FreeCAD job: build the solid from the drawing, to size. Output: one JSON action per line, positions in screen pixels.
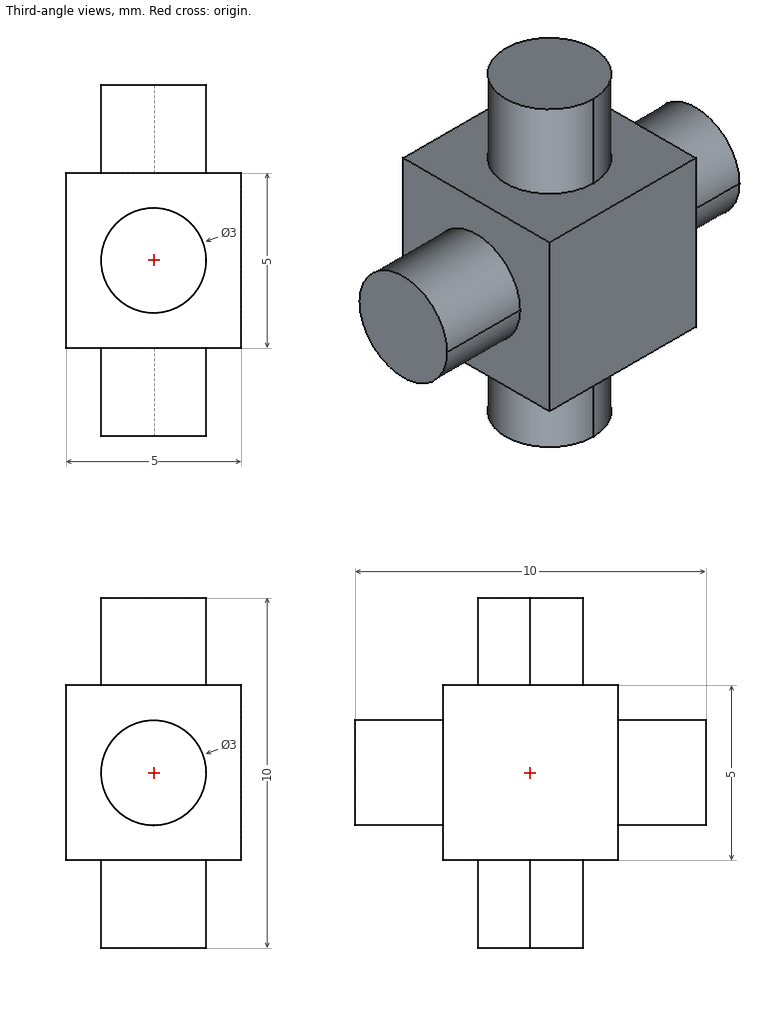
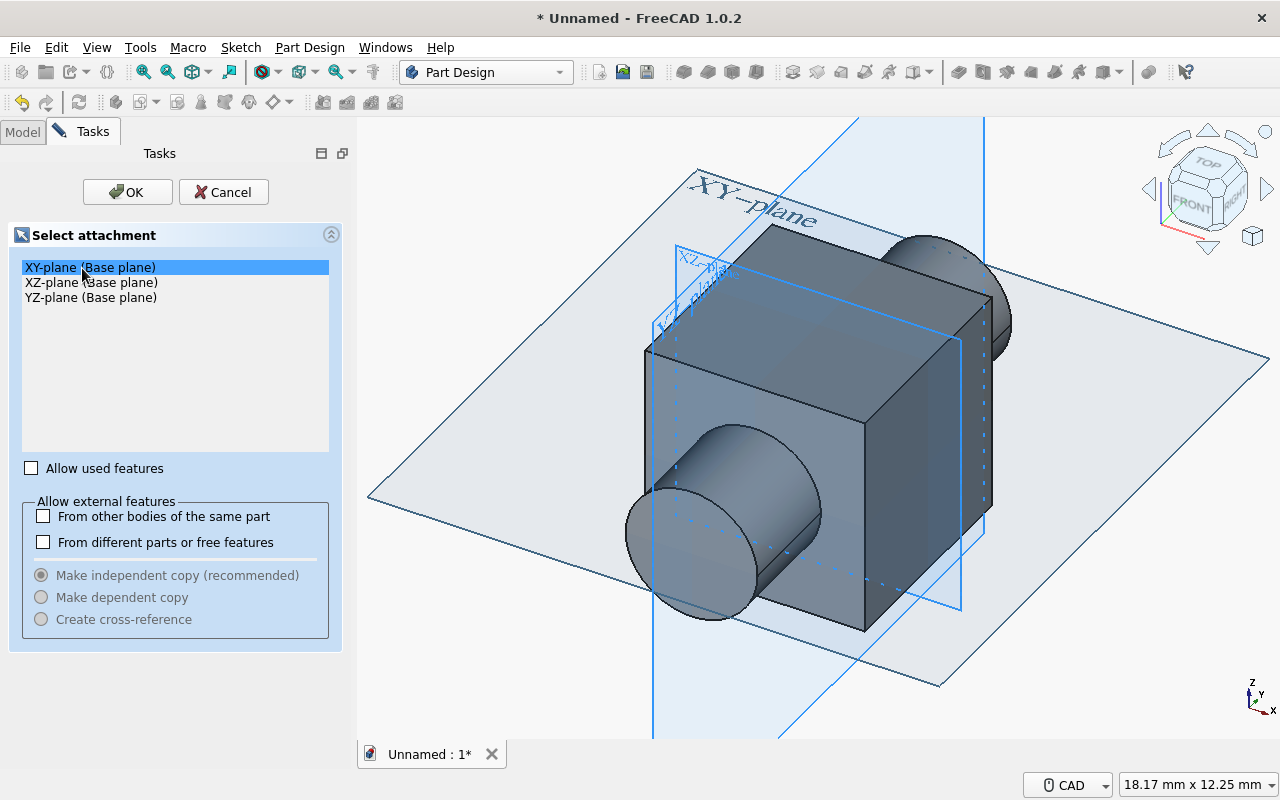
{"action": "left_click", "coordinate": [128, 192]}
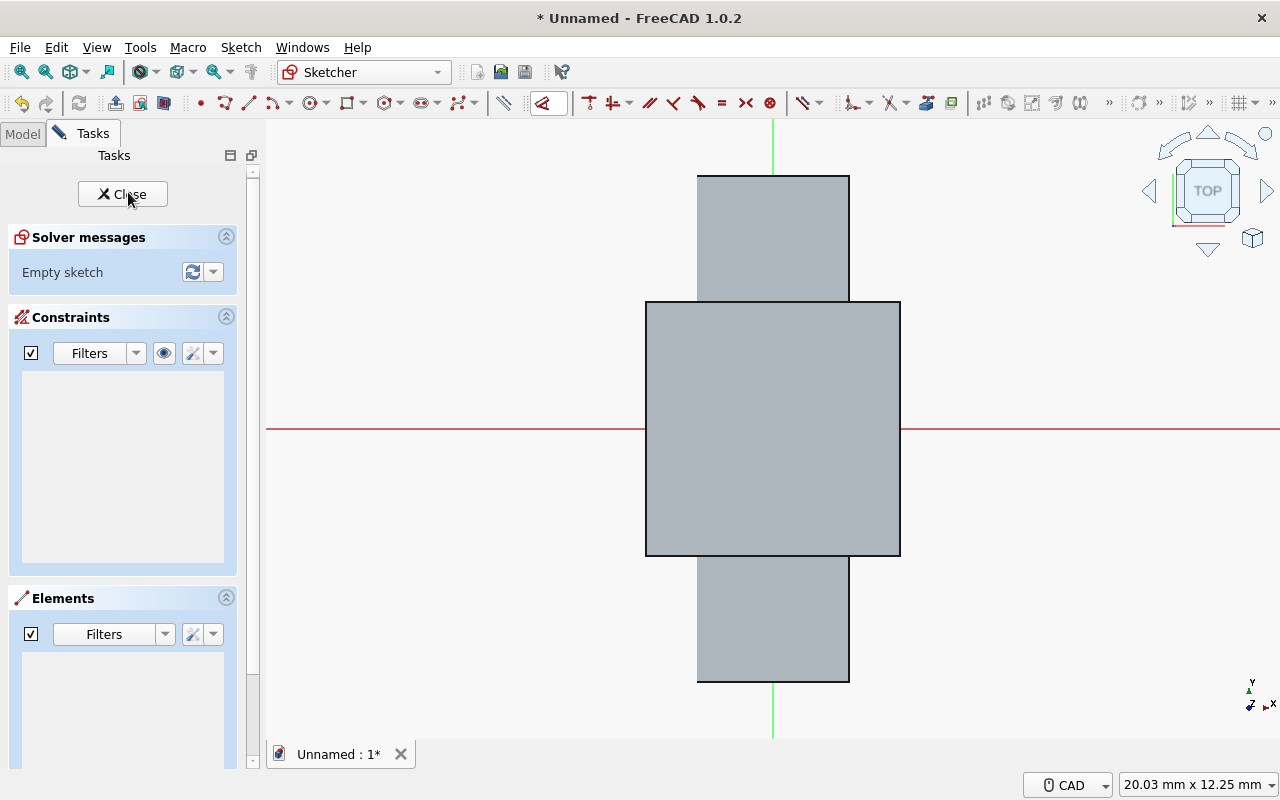
{"action": "left_click", "coordinate": [164, 104]}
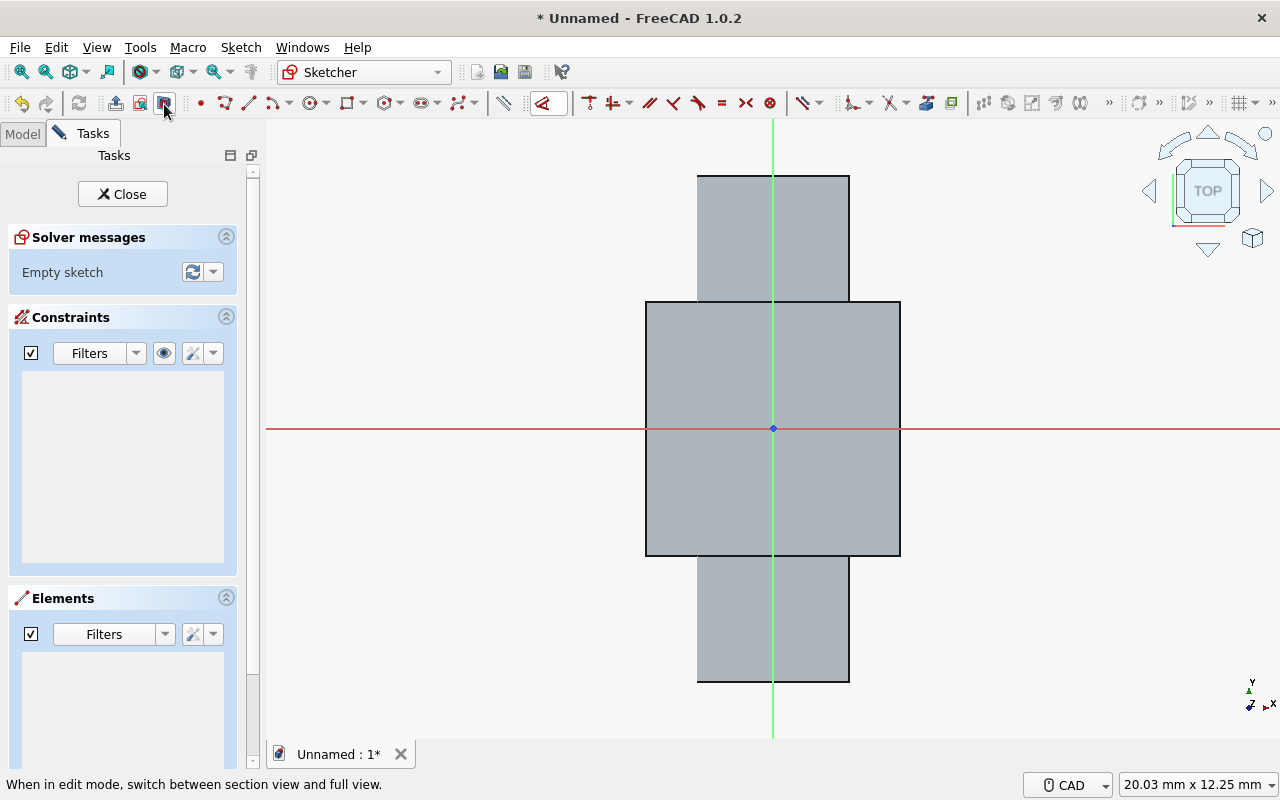
{"action": "scroll", "coordinate": [813, 429], "scroll_direction": "up", "scroll_amount": 5}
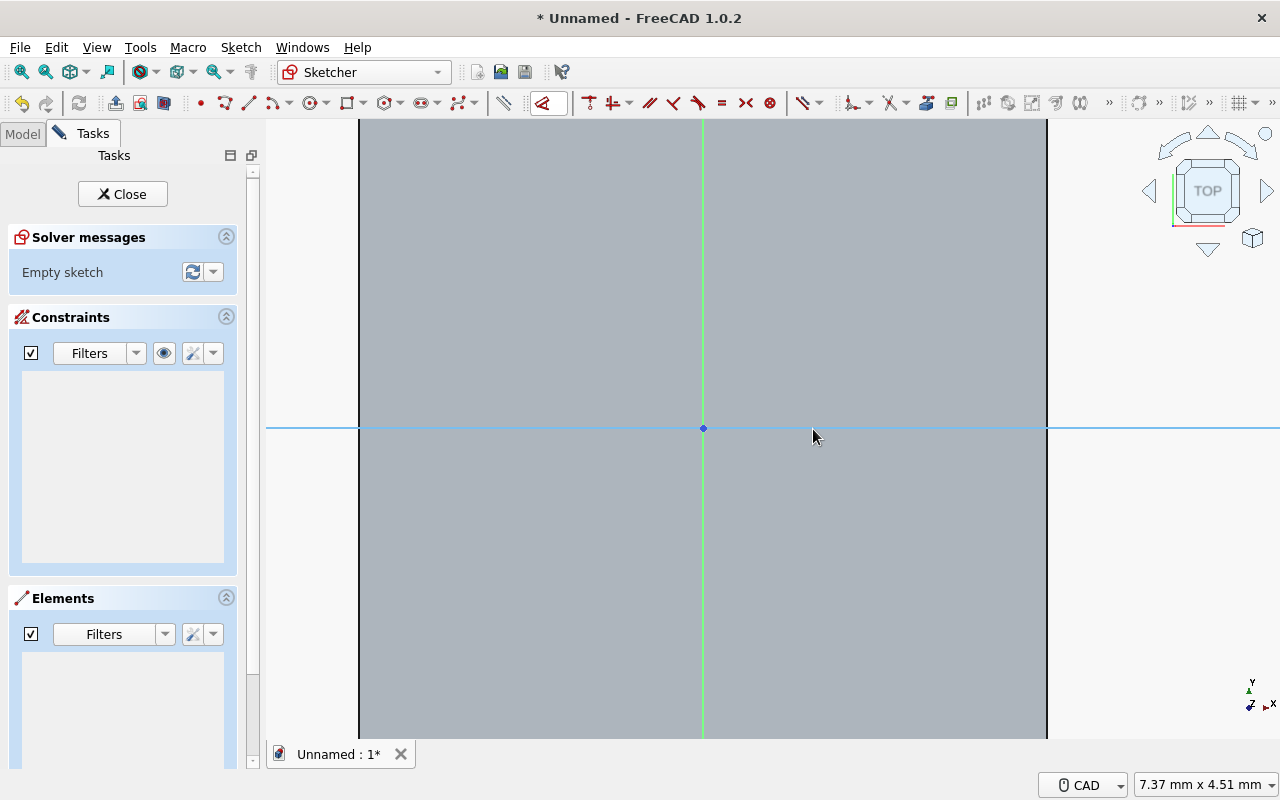
{"action": "left_click", "coordinate": [310, 104]}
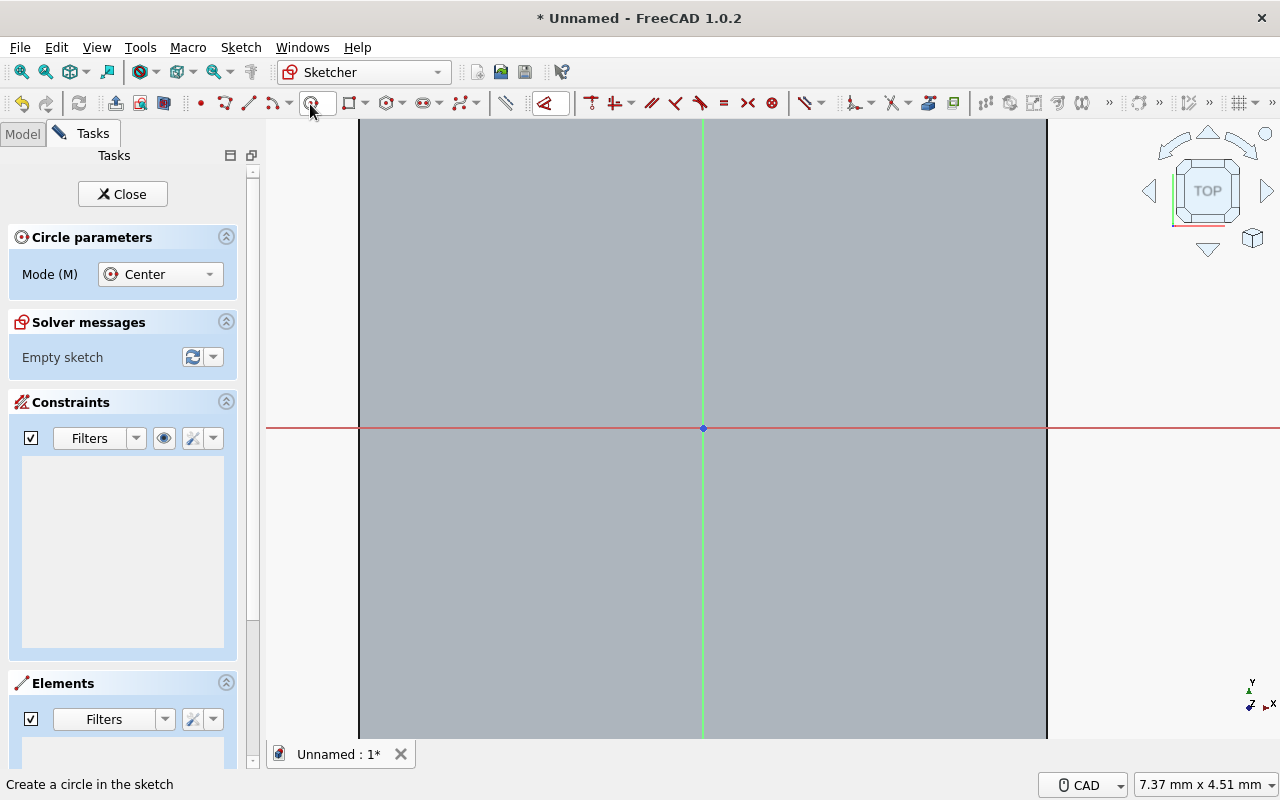
{"action": "left_click", "coordinate": [703, 428]}
{"action": "mouse_move", "coordinate": [849, 282]}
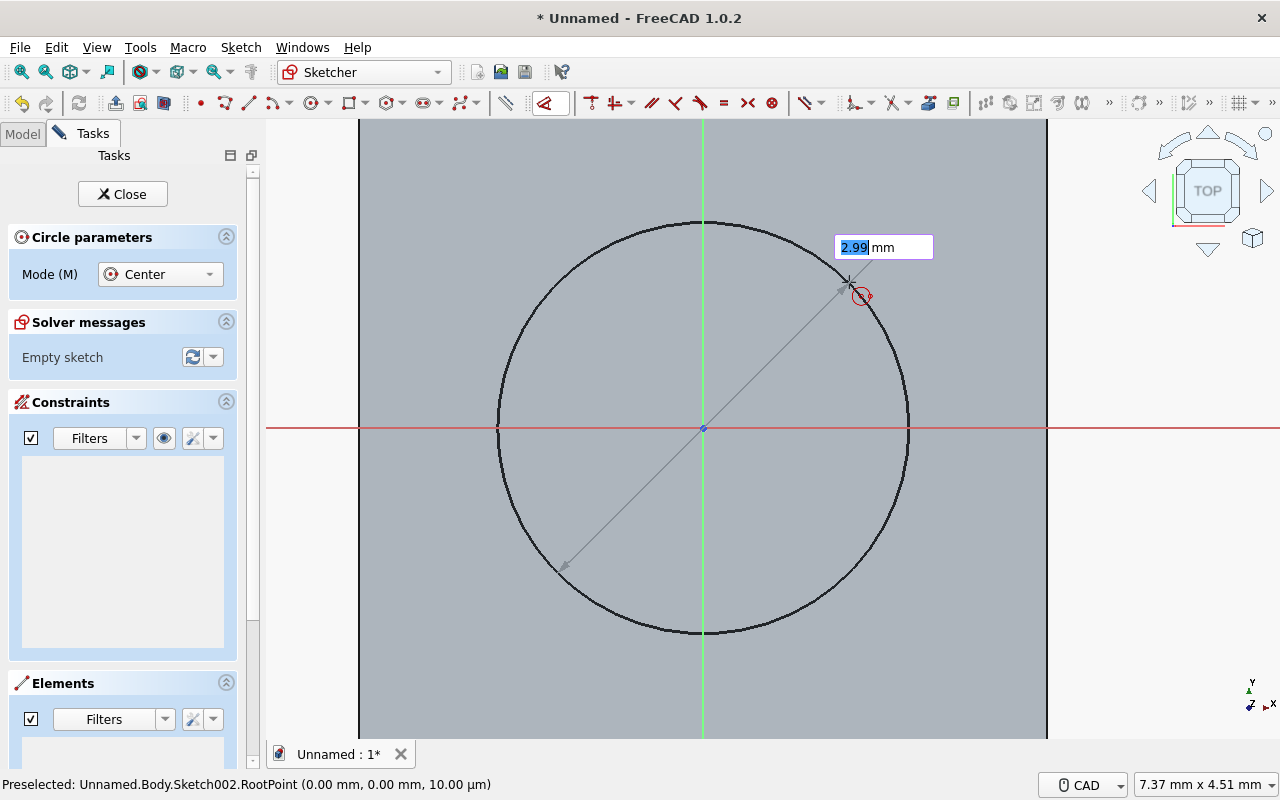
{"action": "type", "text": "3"}
{"action": "key", "text": "Return"}
{"action": "key", "text": "Escape"}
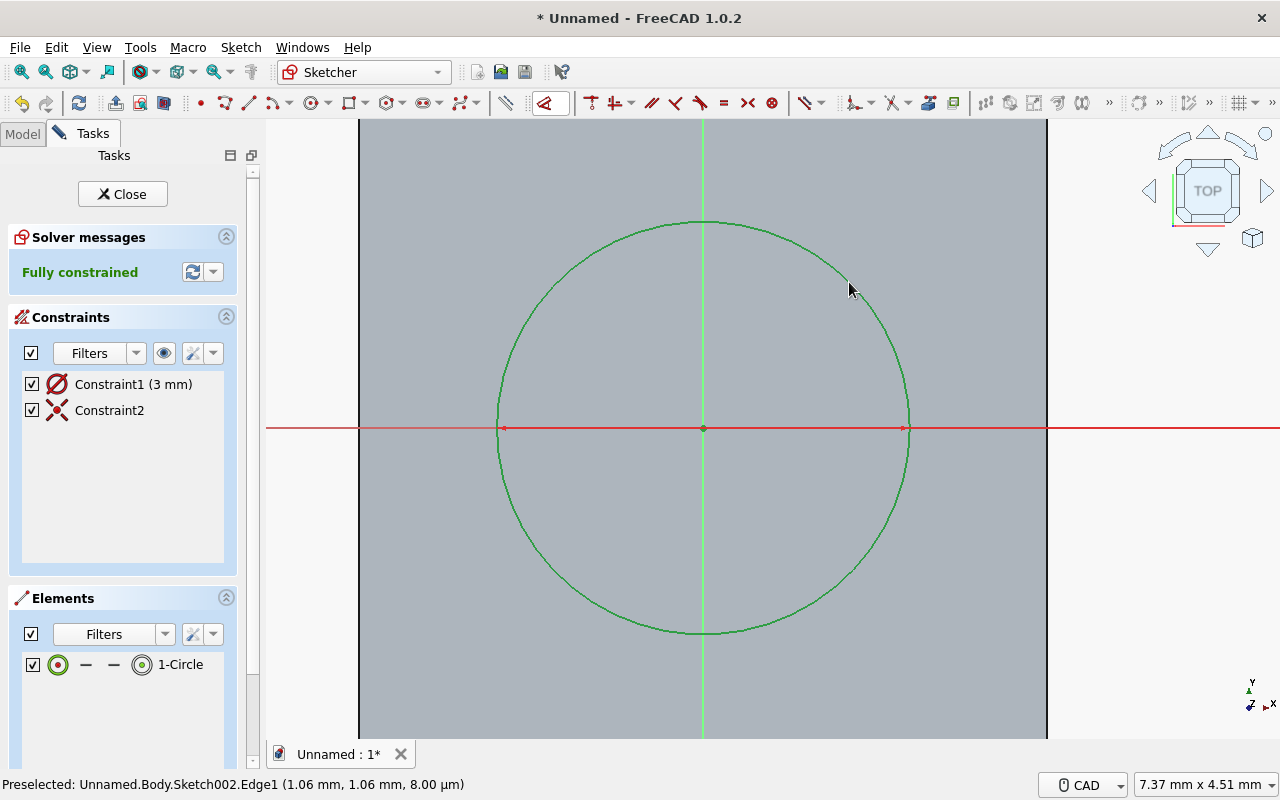
{"action": "left_click", "coordinate": [123, 194]}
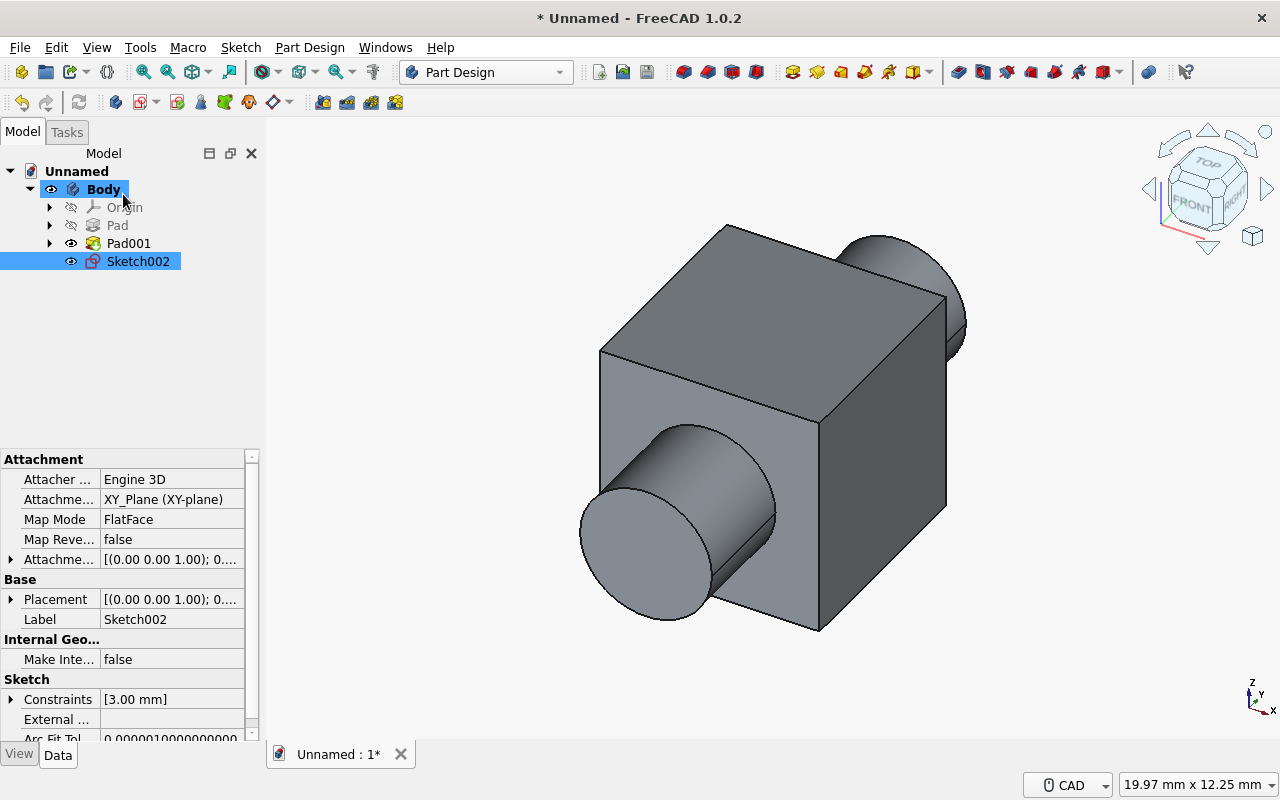
{"action": "left_click", "coordinate": [794, 72]}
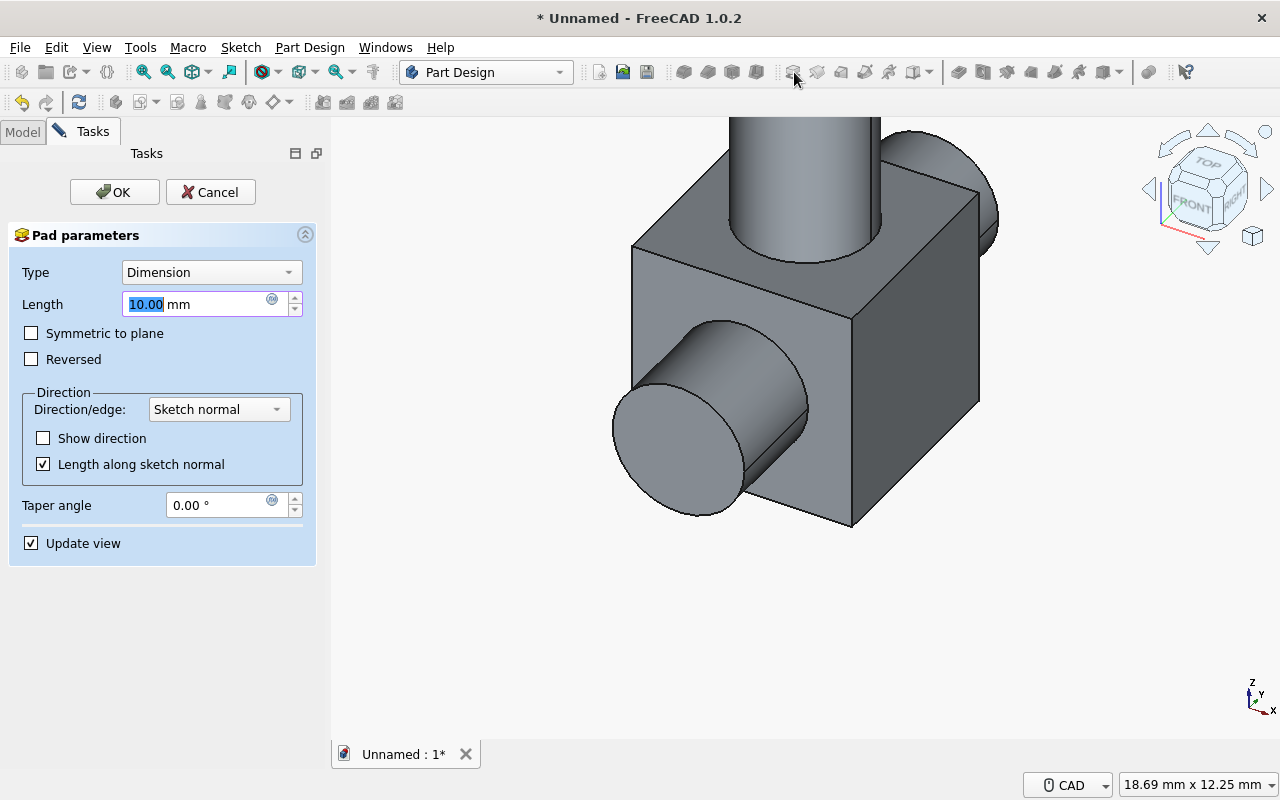
{"action": "type", "text": "10"}
{"action": "key", "text": "Tab"}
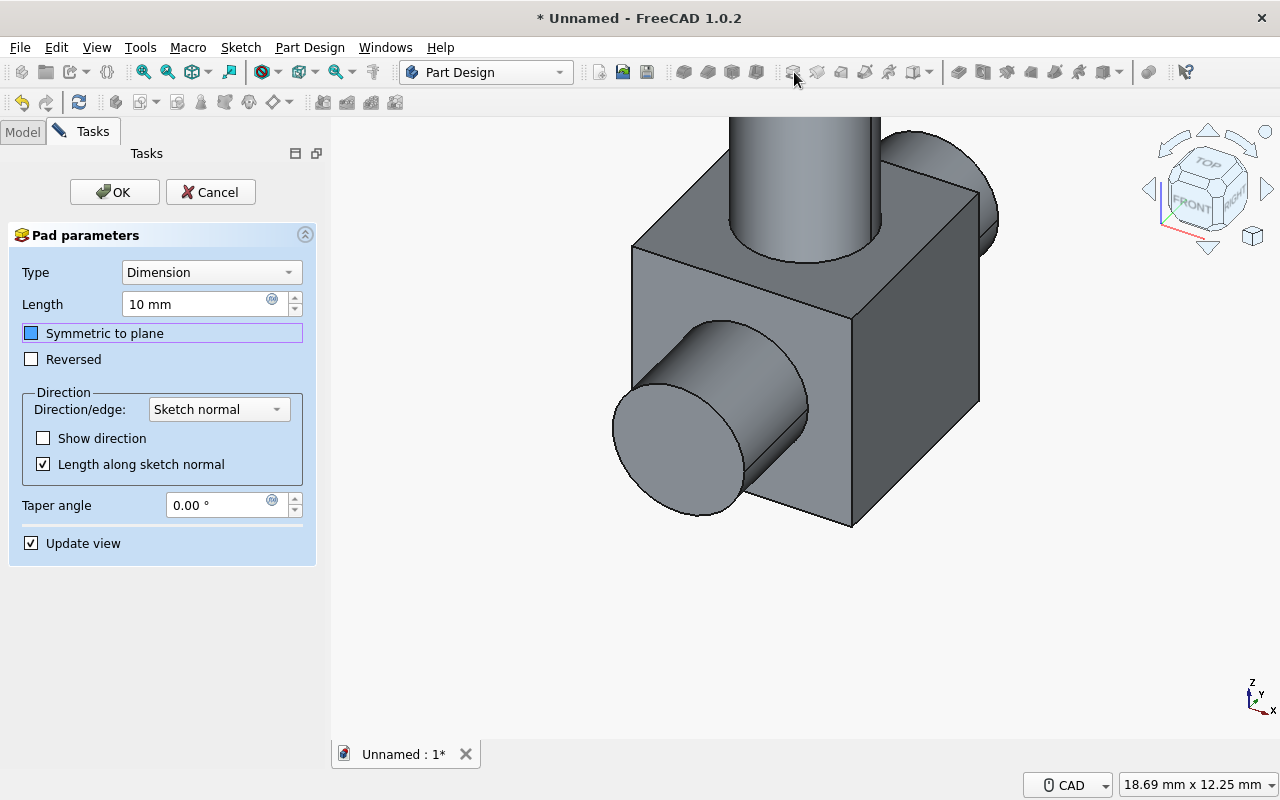
{"action": "left_click", "coordinate": [30, 333]}